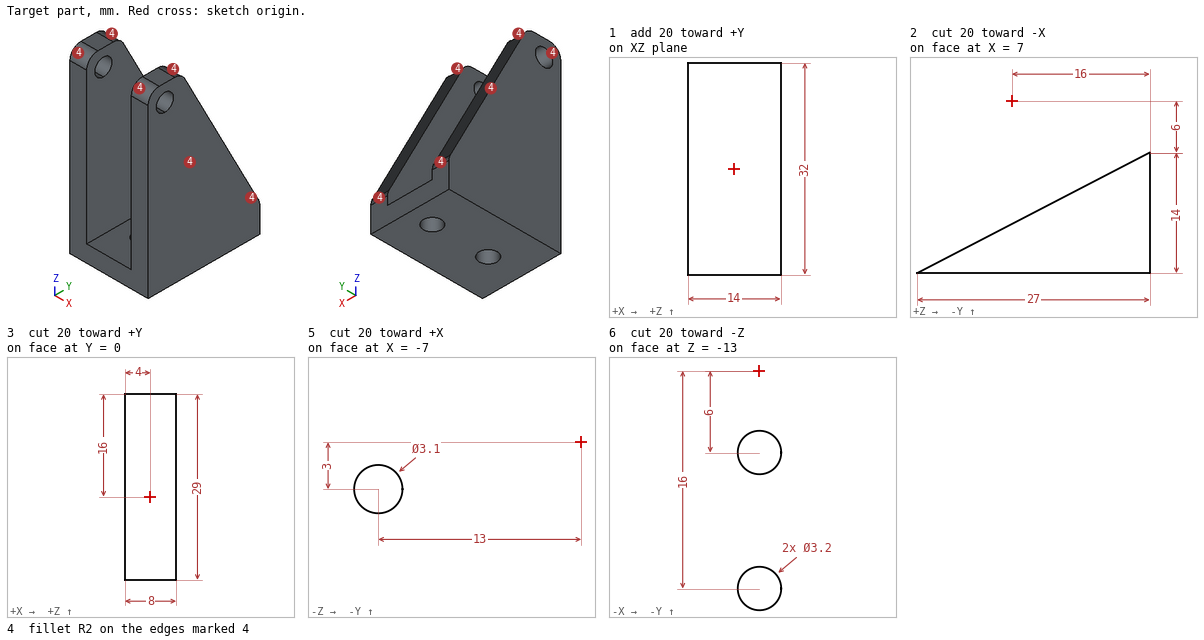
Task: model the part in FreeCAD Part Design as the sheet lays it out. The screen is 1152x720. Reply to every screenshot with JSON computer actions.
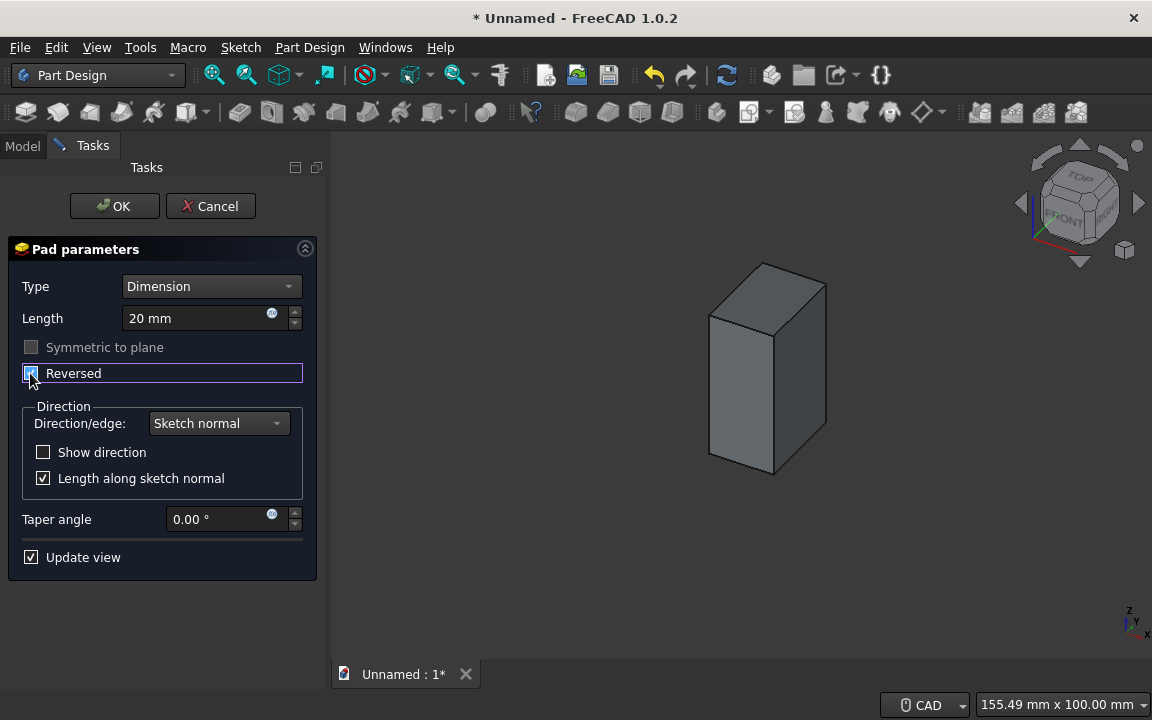
{"action": "left_click", "coordinate": [115, 206]}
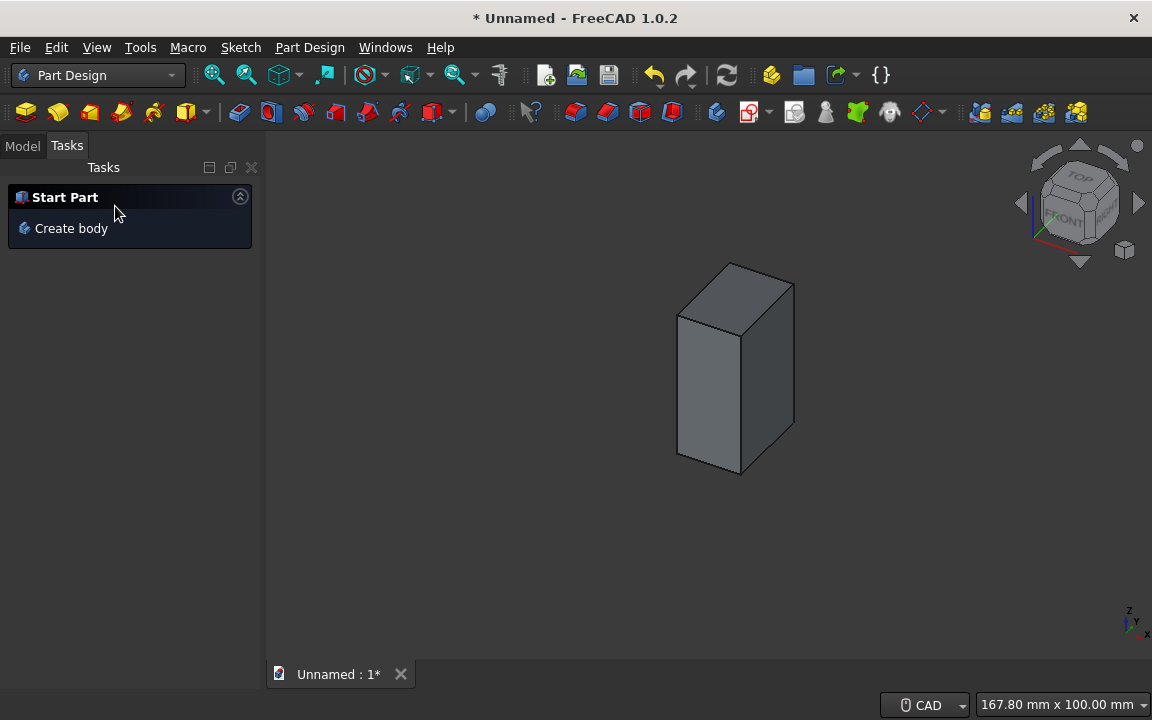
{"action": "left_click", "coordinate": [216, 76]}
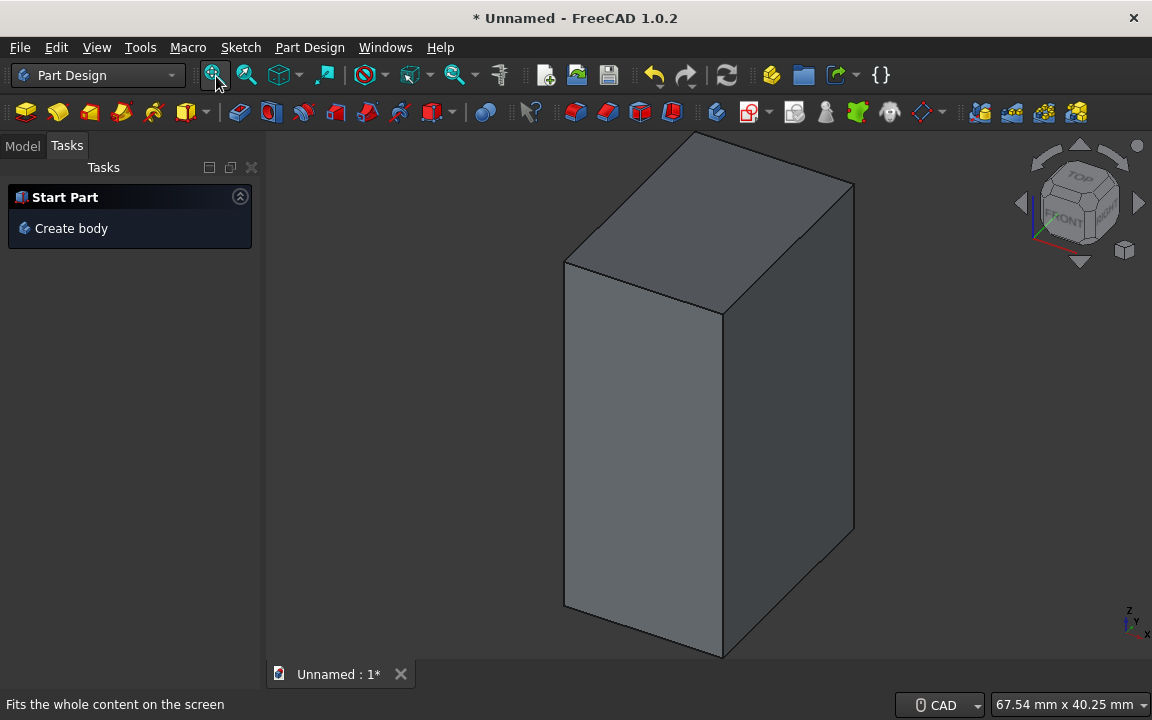
{"action": "left_click", "coordinate": [789, 420]}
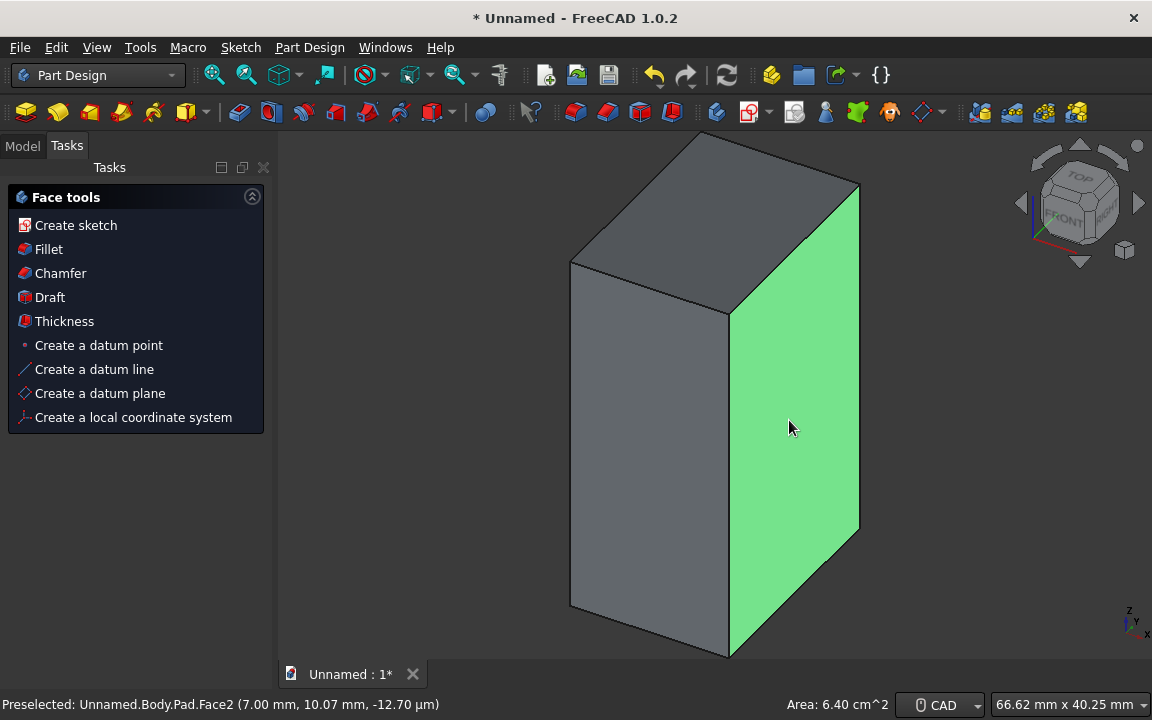
{"action": "left_click", "coordinate": [750, 112]}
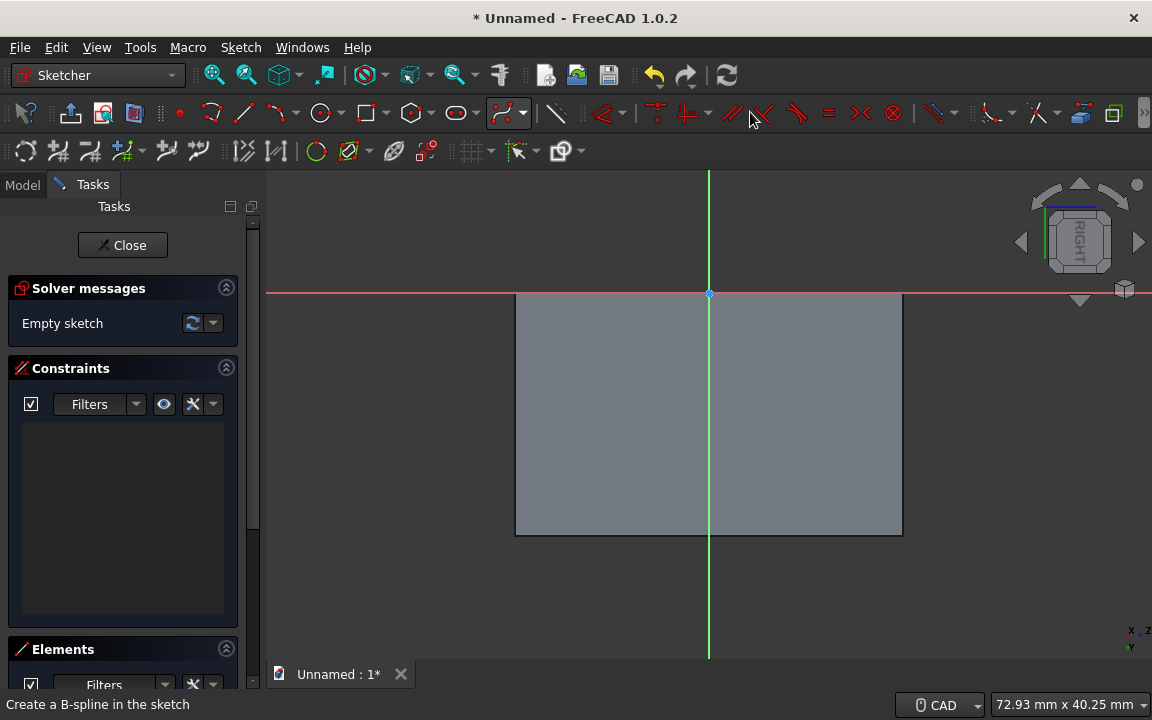
{"action": "left_click", "coordinate": [212, 114]}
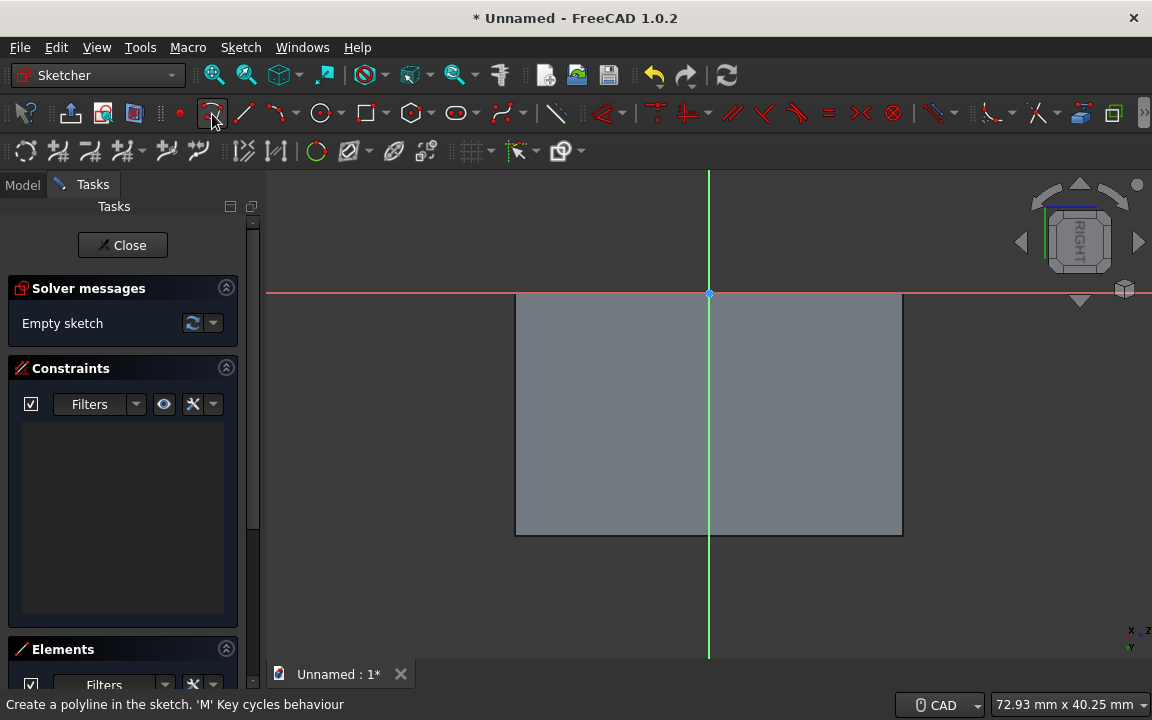
{"action": "left_click", "coordinate": [903, 366]}
{"action": "left_click", "coordinate": [575, 536]}
{"action": "left_click", "coordinate": [903, 536]}
{"action": "left_click", "coordinate": [903, 367]}
{"action": "key", "text": "Escape"}
{"action": "key", "text": "Escape"}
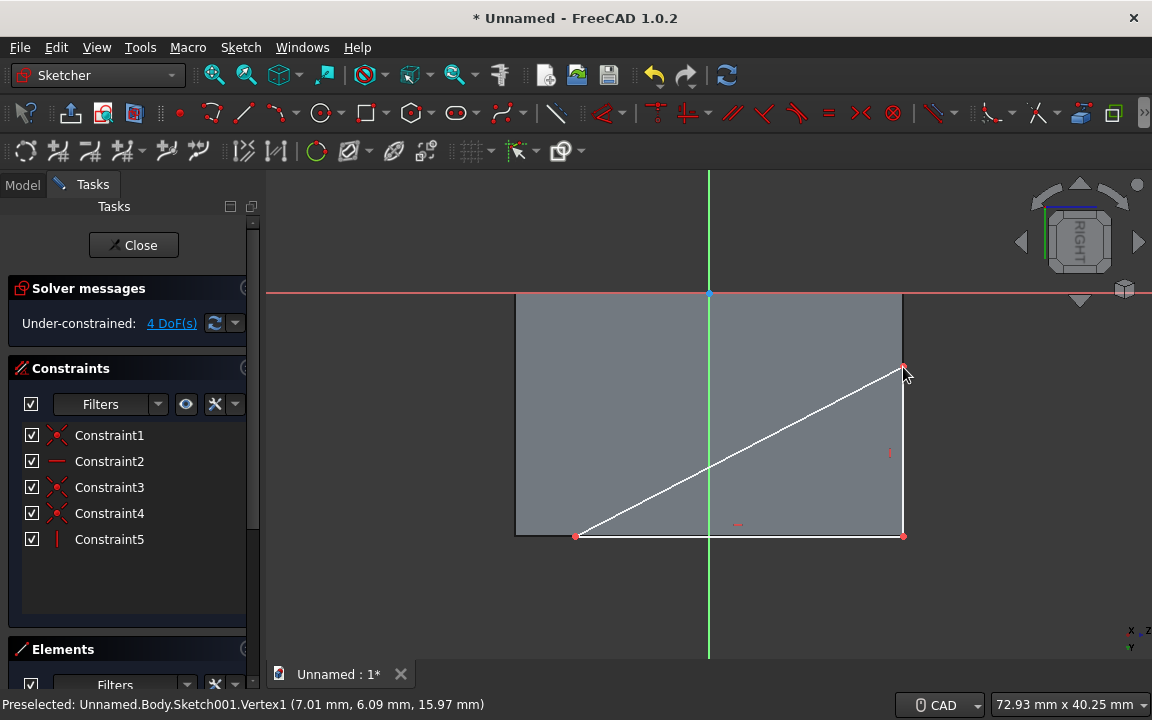
{"action": "key", "text": "d"}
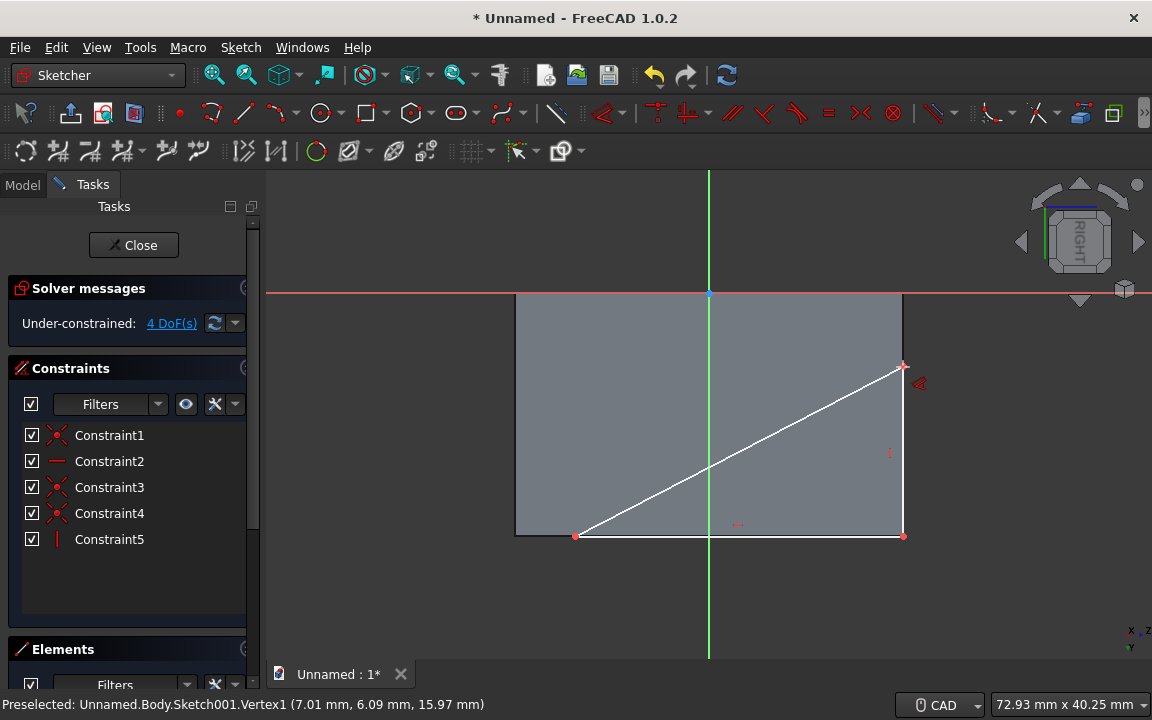
{"action": "left_click", "coordinate": [673, 537]}
{"action": "left_click", "coordinate": [739, 571]}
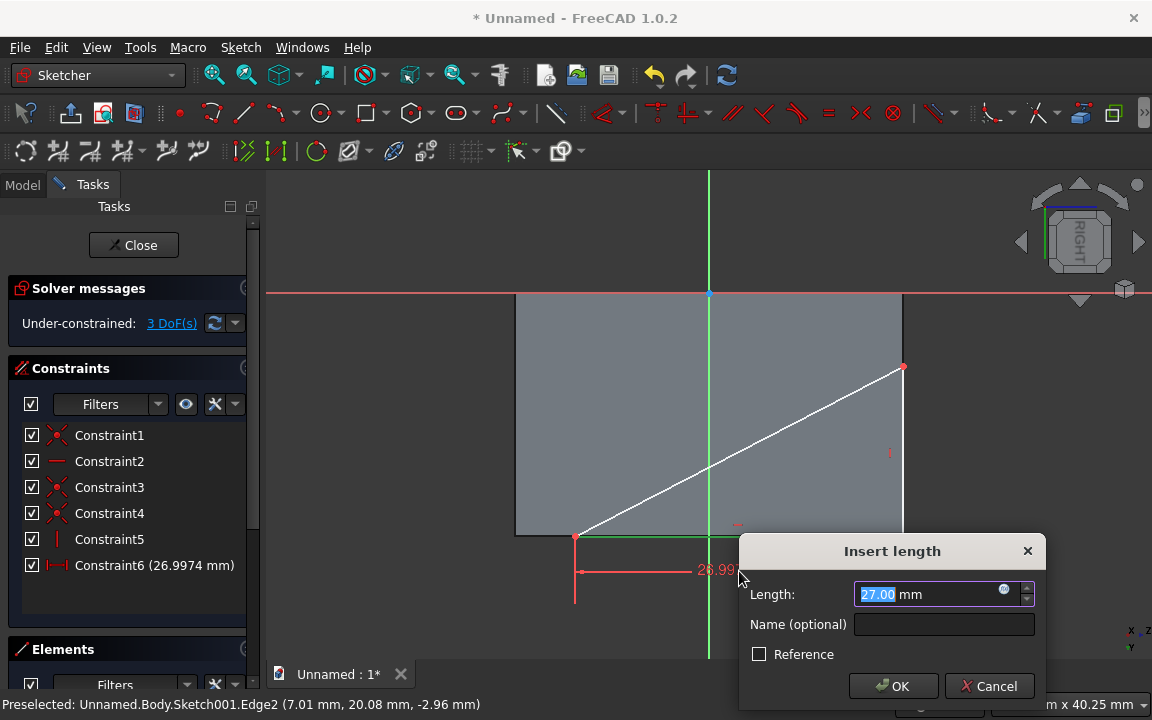
{"action": "type", "text": "27"}
{"action": "key", "text": "Return"}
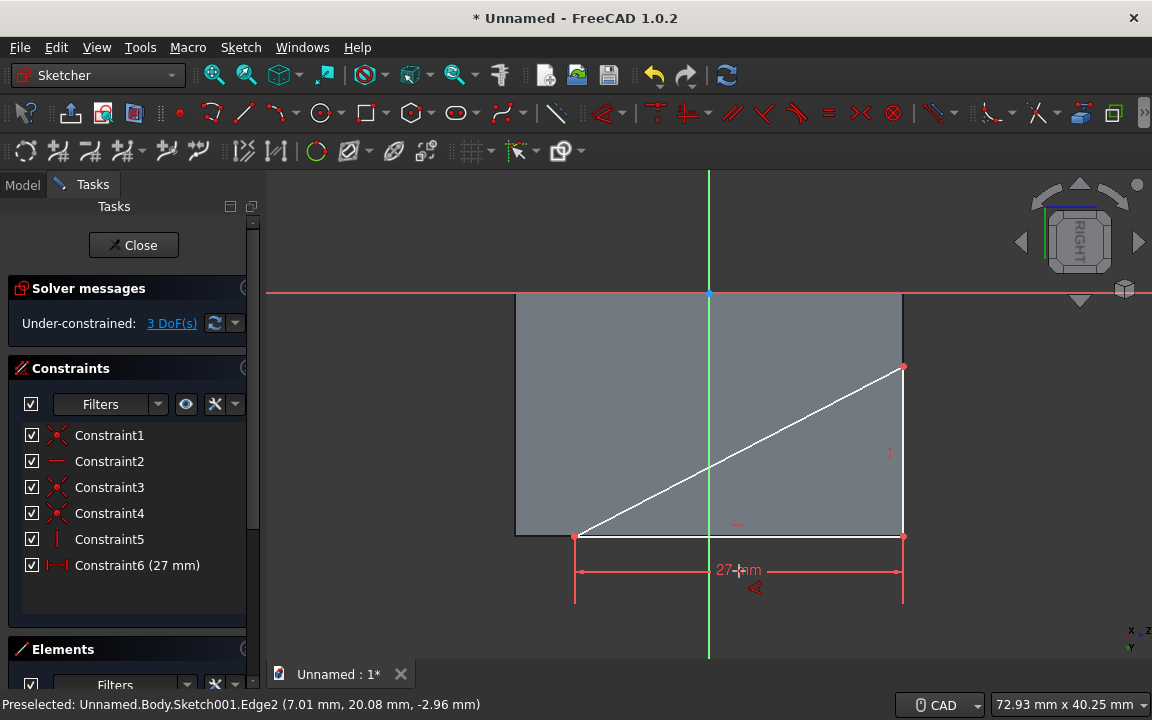
{"action": "left_click", "coordinate": [903, 486]}
{"action": "left_click", "coordinate": [937, 452]}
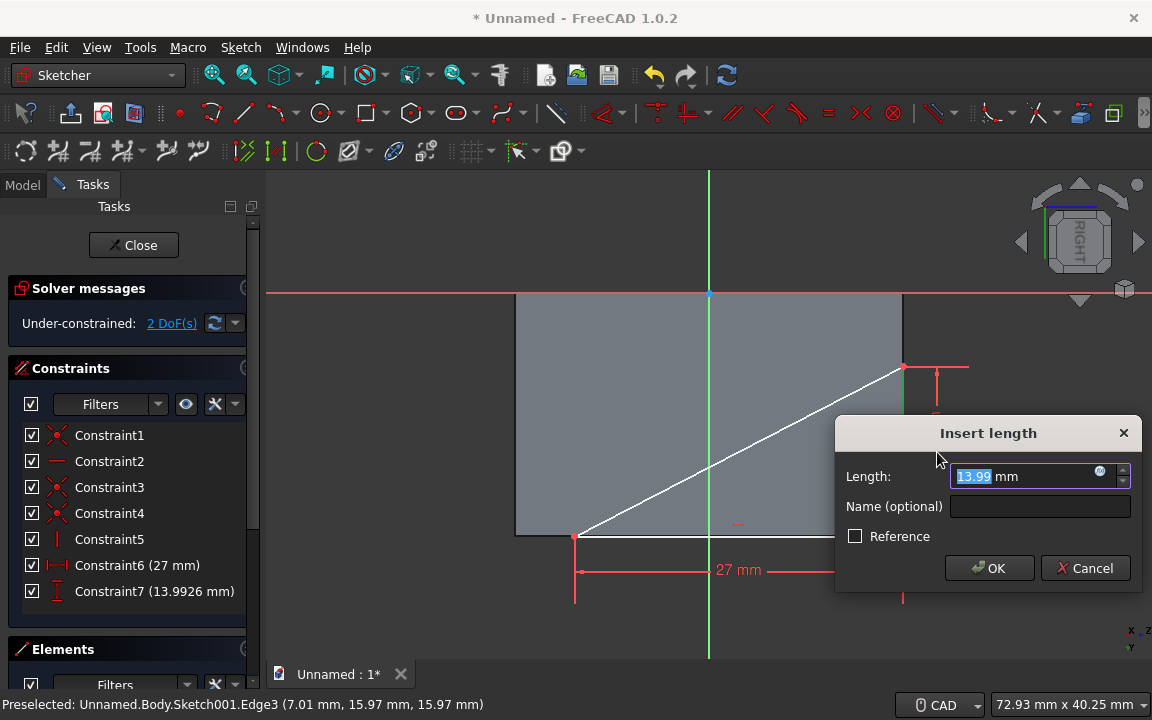
{"action": "type", "text": "14"}
{"action": "key", "text": "Return"}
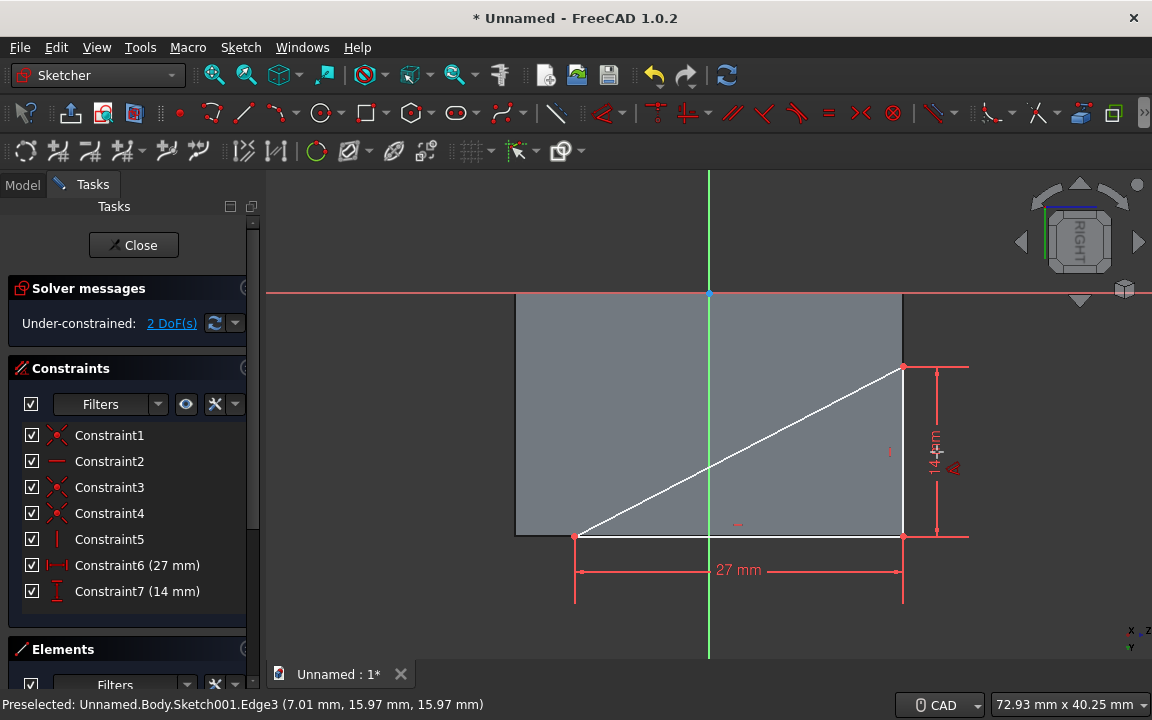
{"action": "left_click", "coordinate": [903, 367]}
{"action": "left_click", "coordinate": [937, 330]}